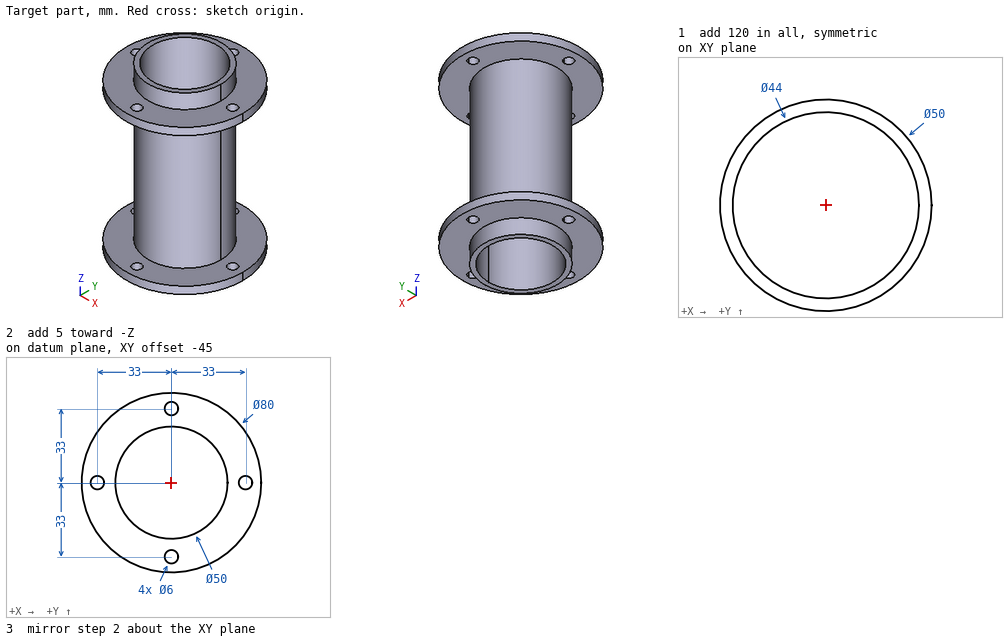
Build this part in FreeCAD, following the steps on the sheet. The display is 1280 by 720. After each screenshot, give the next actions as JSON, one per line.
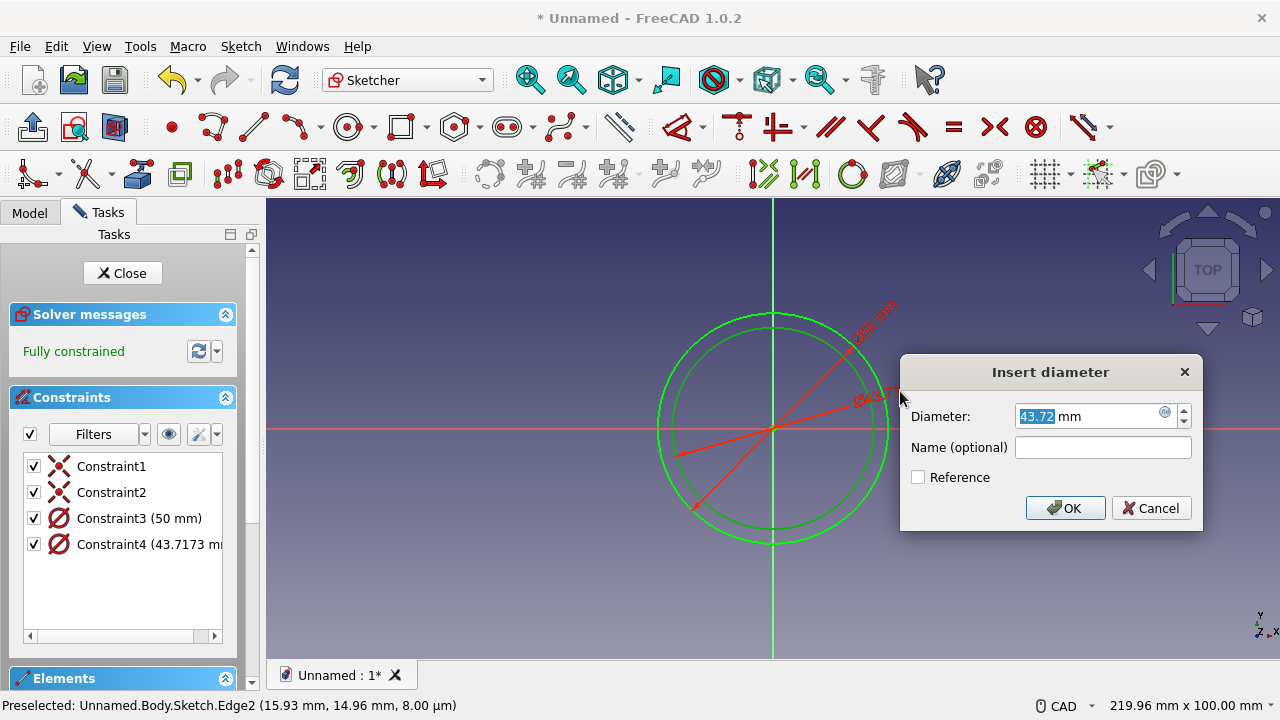
{"action": "type", "text": "44"}
{"action": "key", "text": "Return"}
{"action": "key", "text": "Escape"}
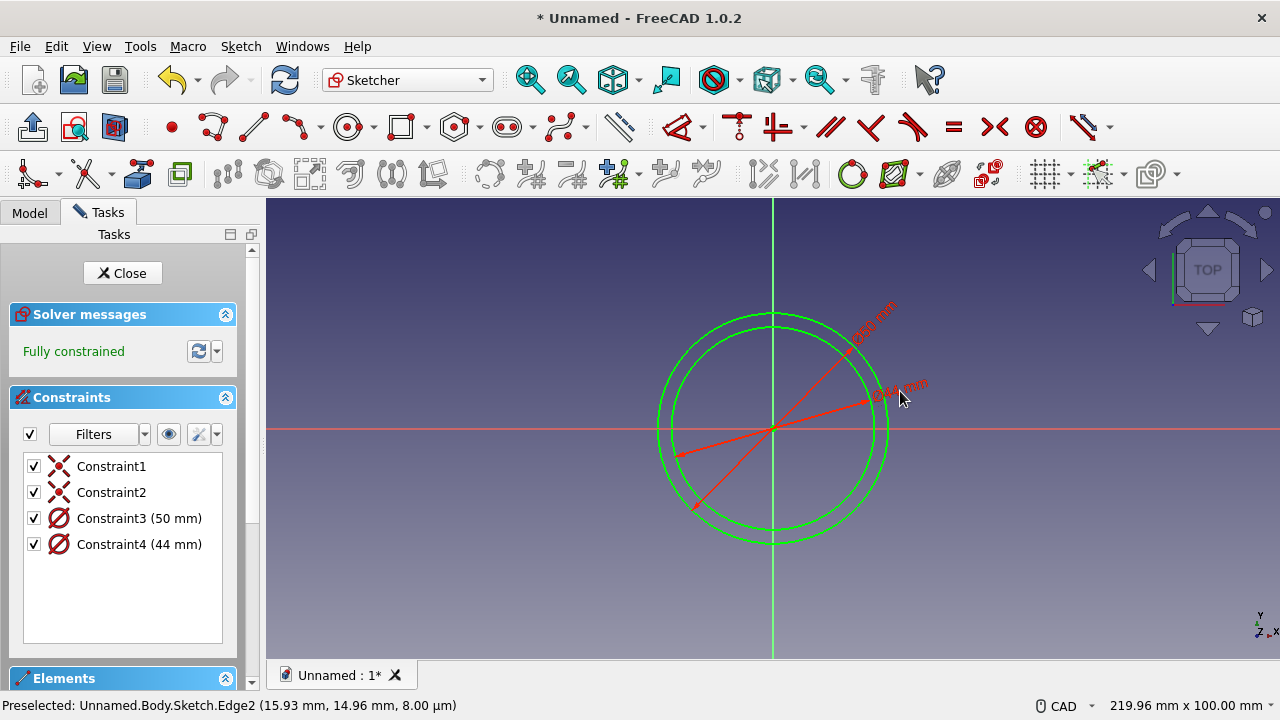
{"action": "left_click", "coordinate": [123, 273]}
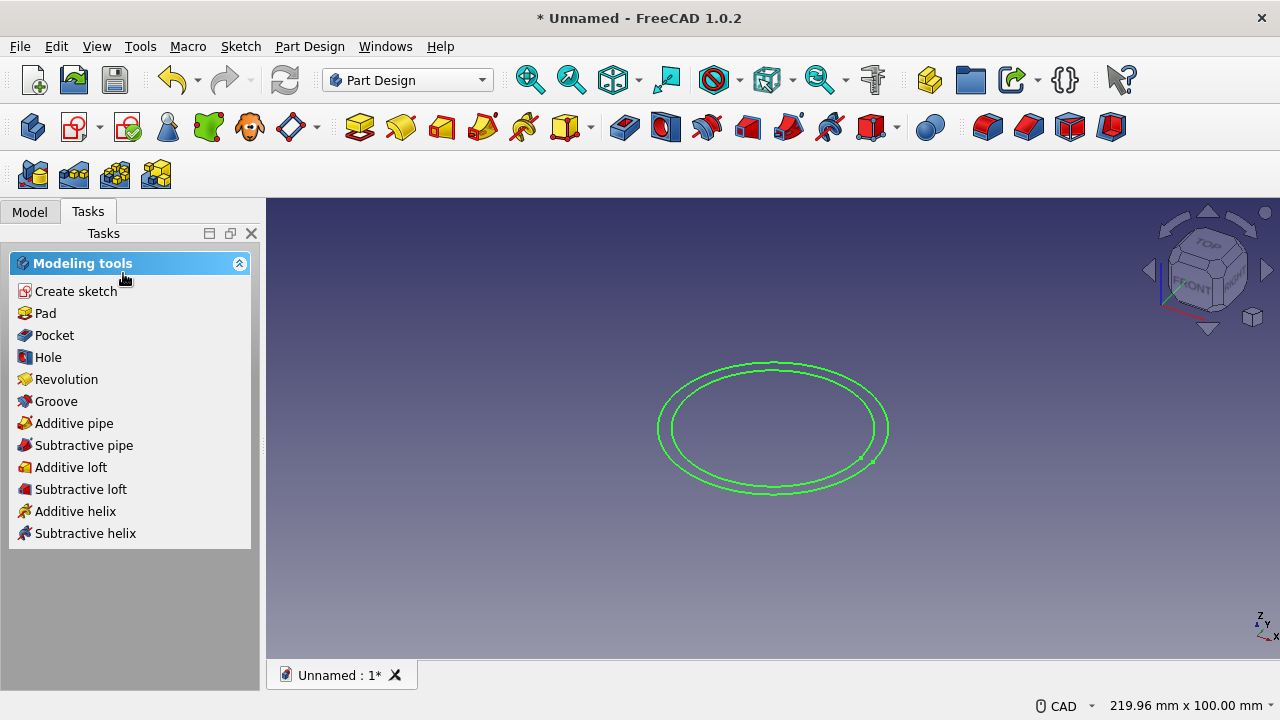
{"action": "left_click", "coordinate": [360, 128]}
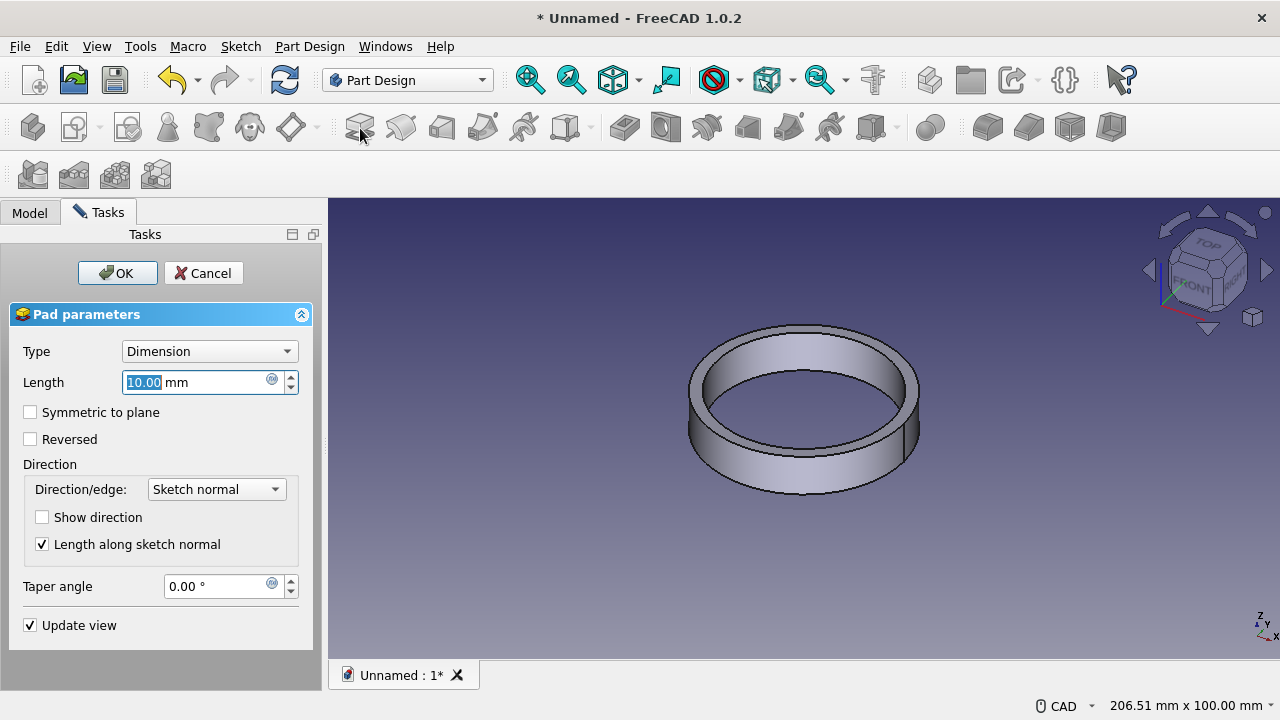
{"action": "type", "text": "120"}
{"action": "key", "text": "Tab"}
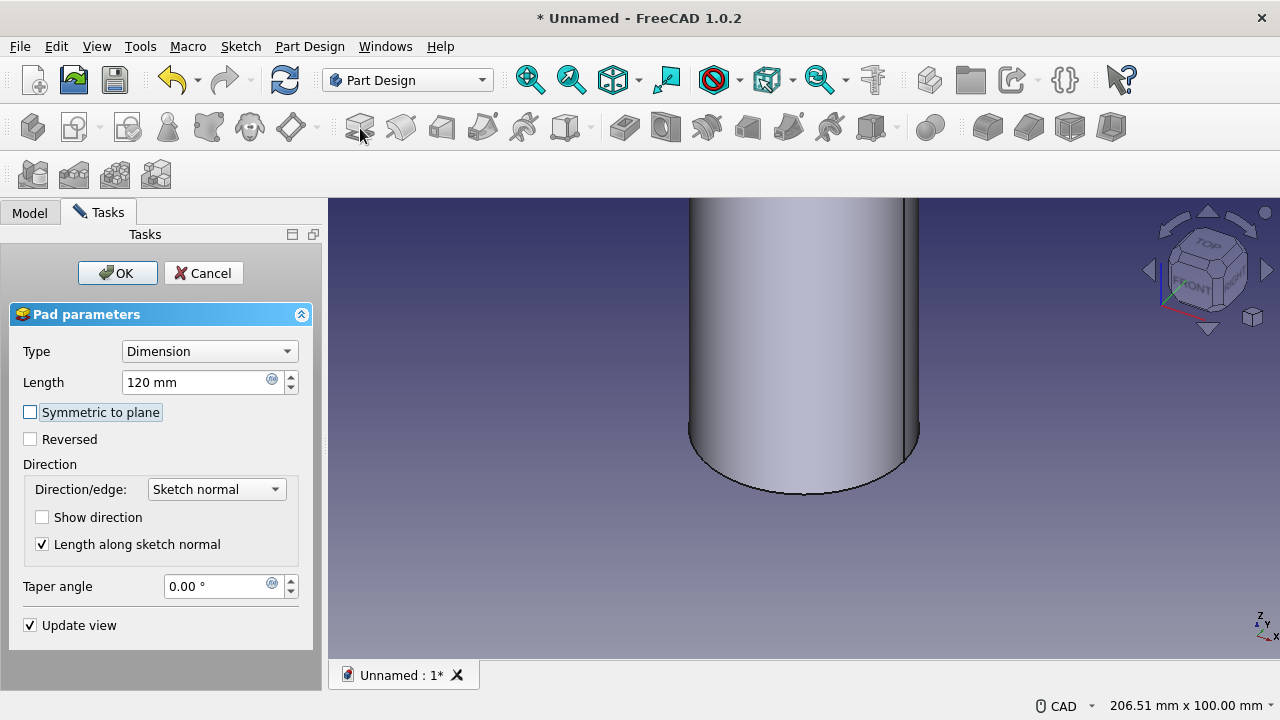
{"action": "left_click", "coordinate": [31, 412]}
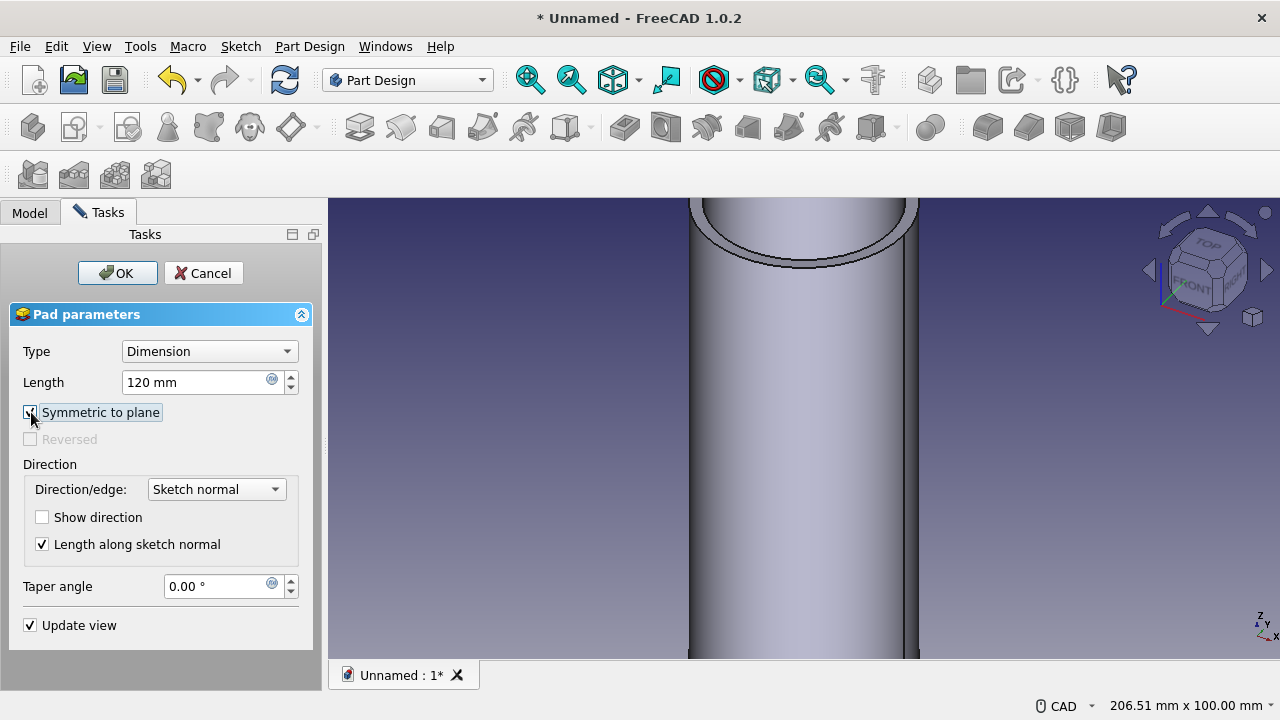
{"action": "left_click", "coordinate": [118, 273]}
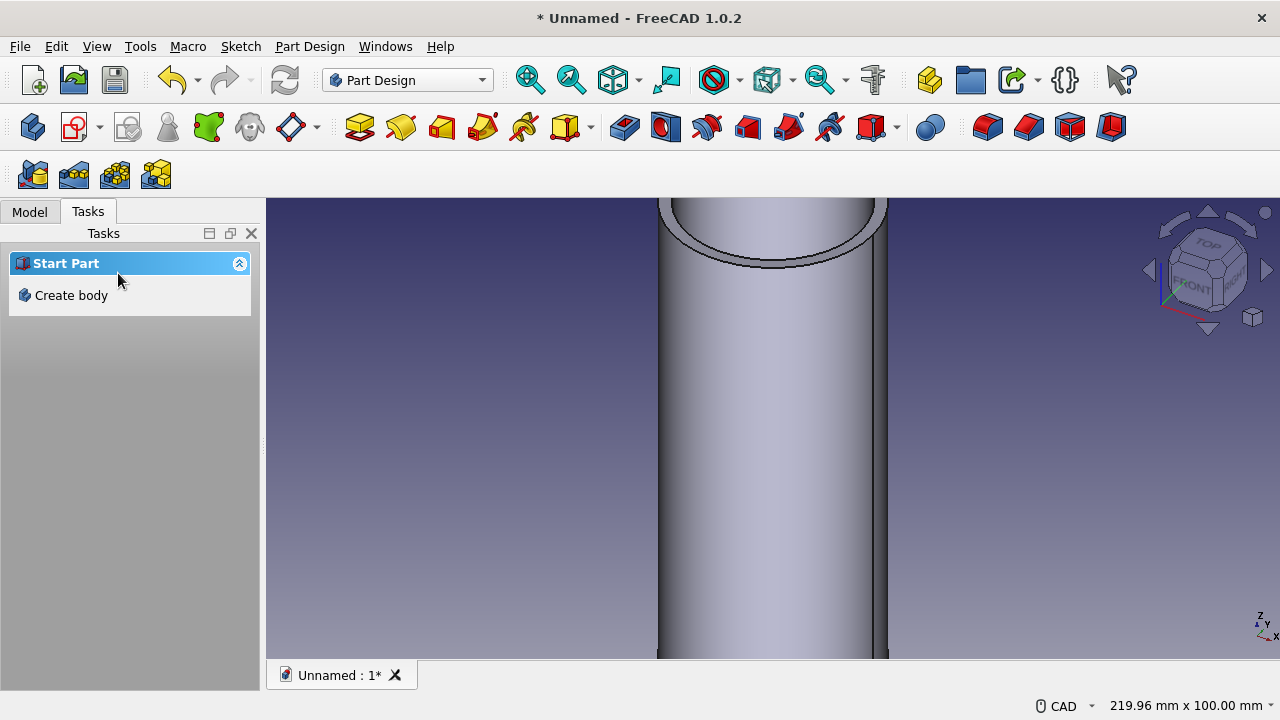
{"action": "left_click", "coordinate": [531, 80]}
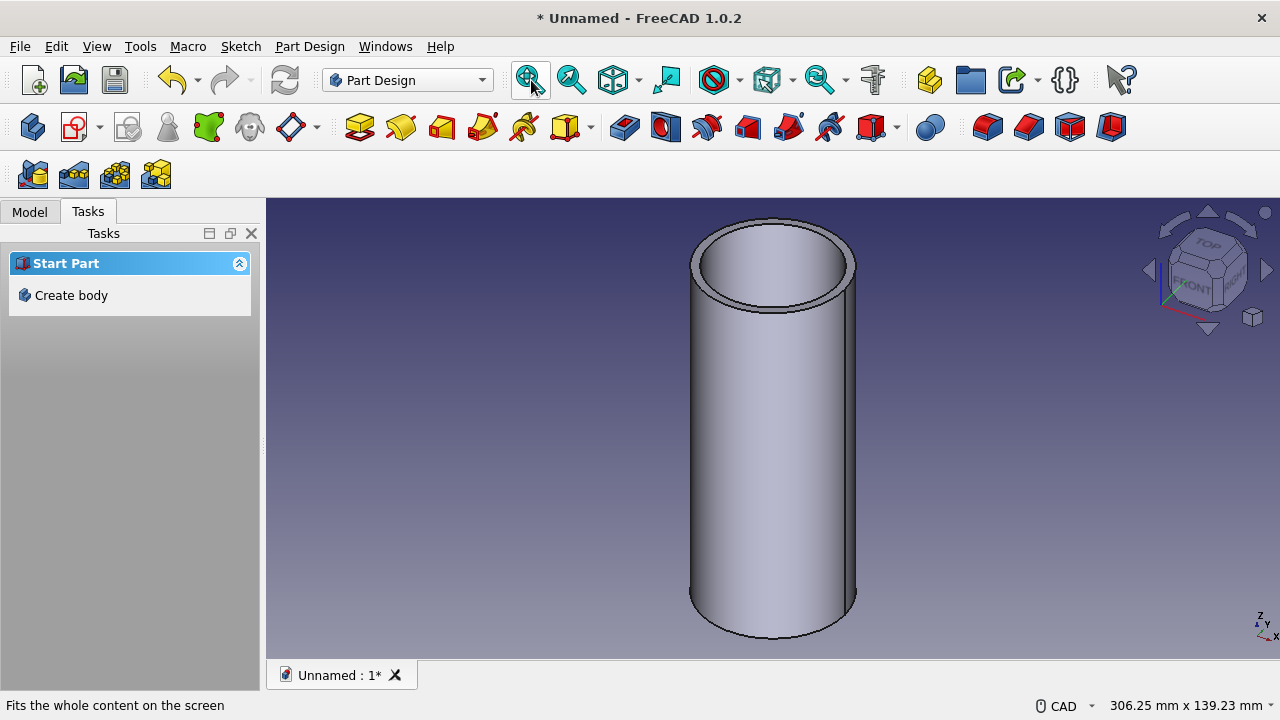
{"action": "left_click", "coordinate": [30, 212]}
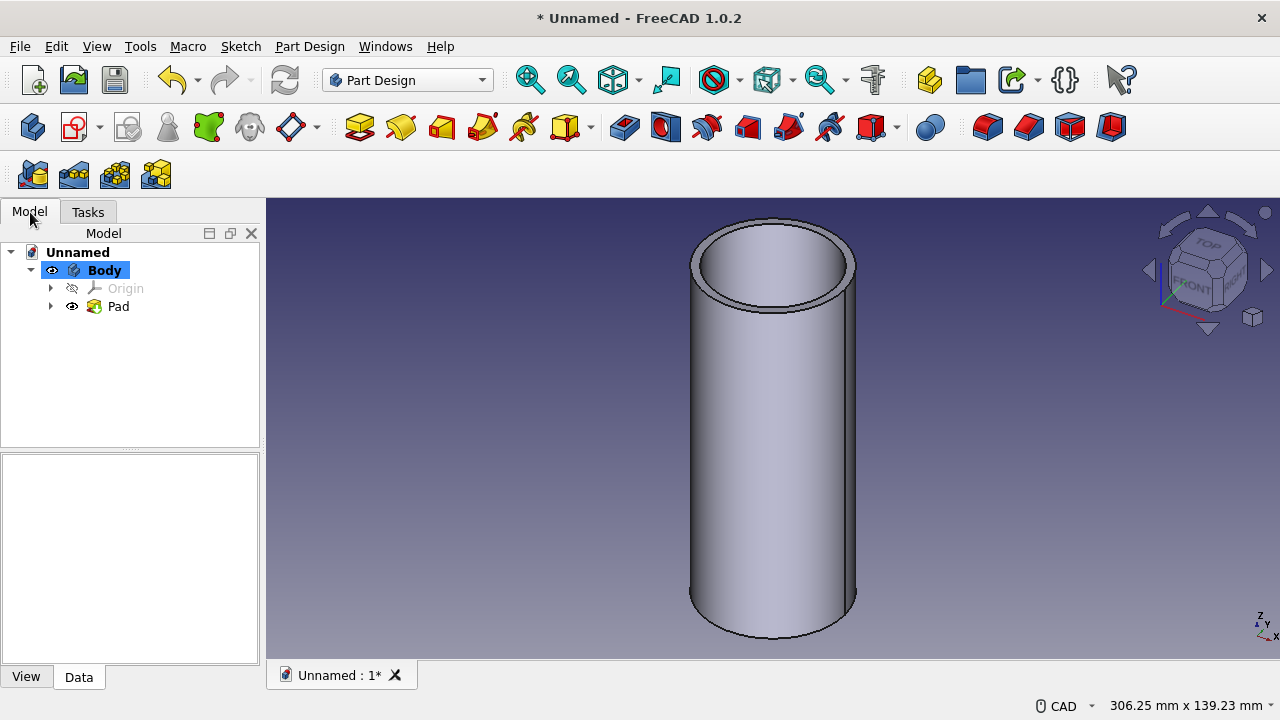
{"action": "left_click", "coordinate": [51, 288]}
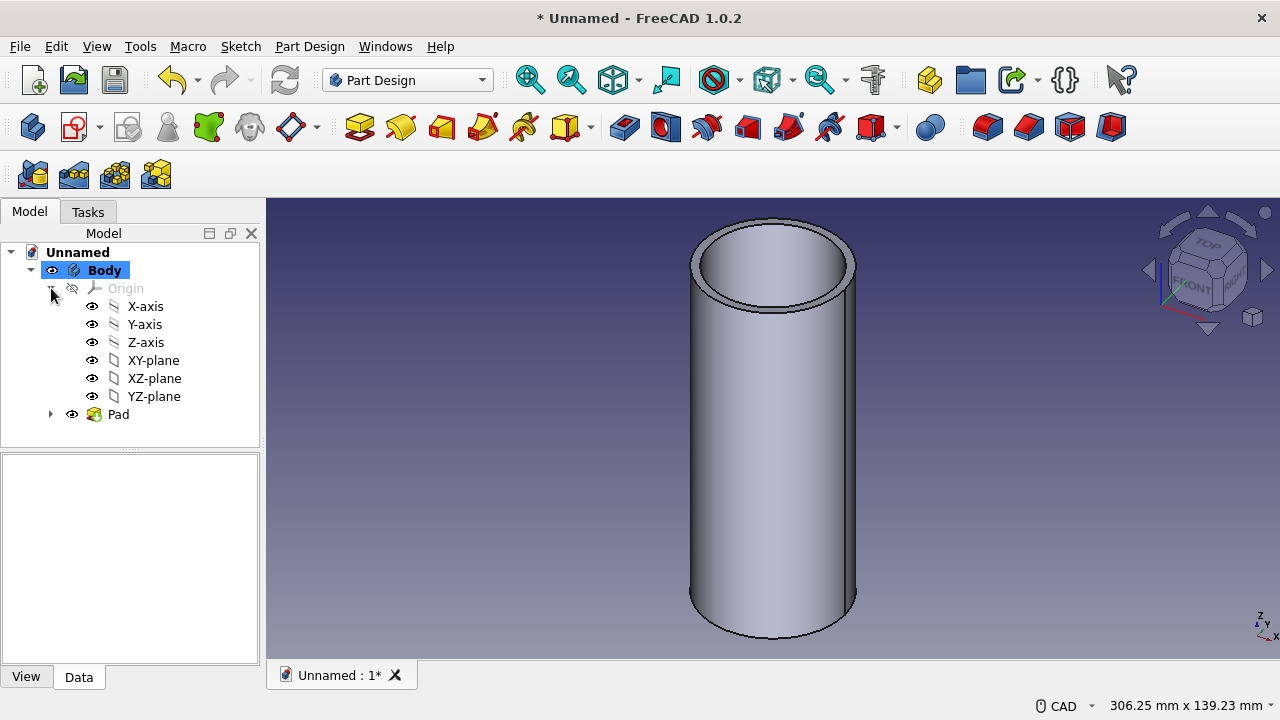
{"action": "left_click", "coordinate": [137, 360]}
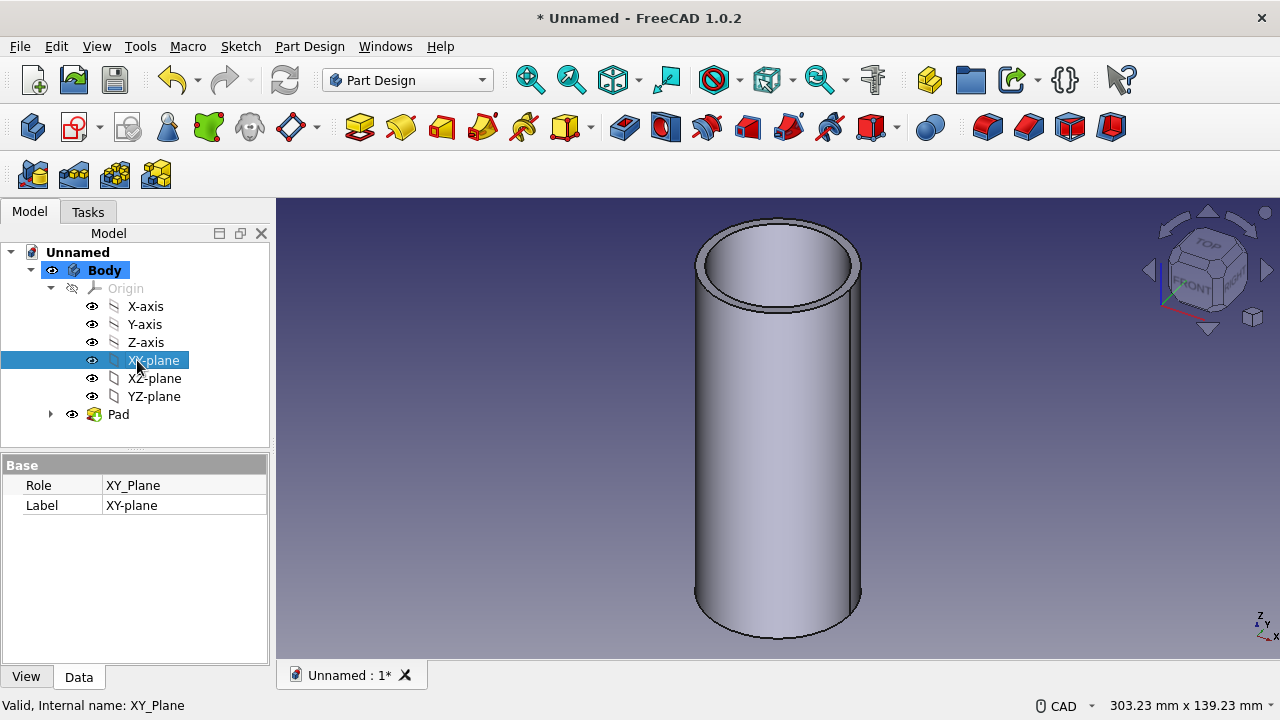
{"action": "left_click", "coordinate": [290, 128]}